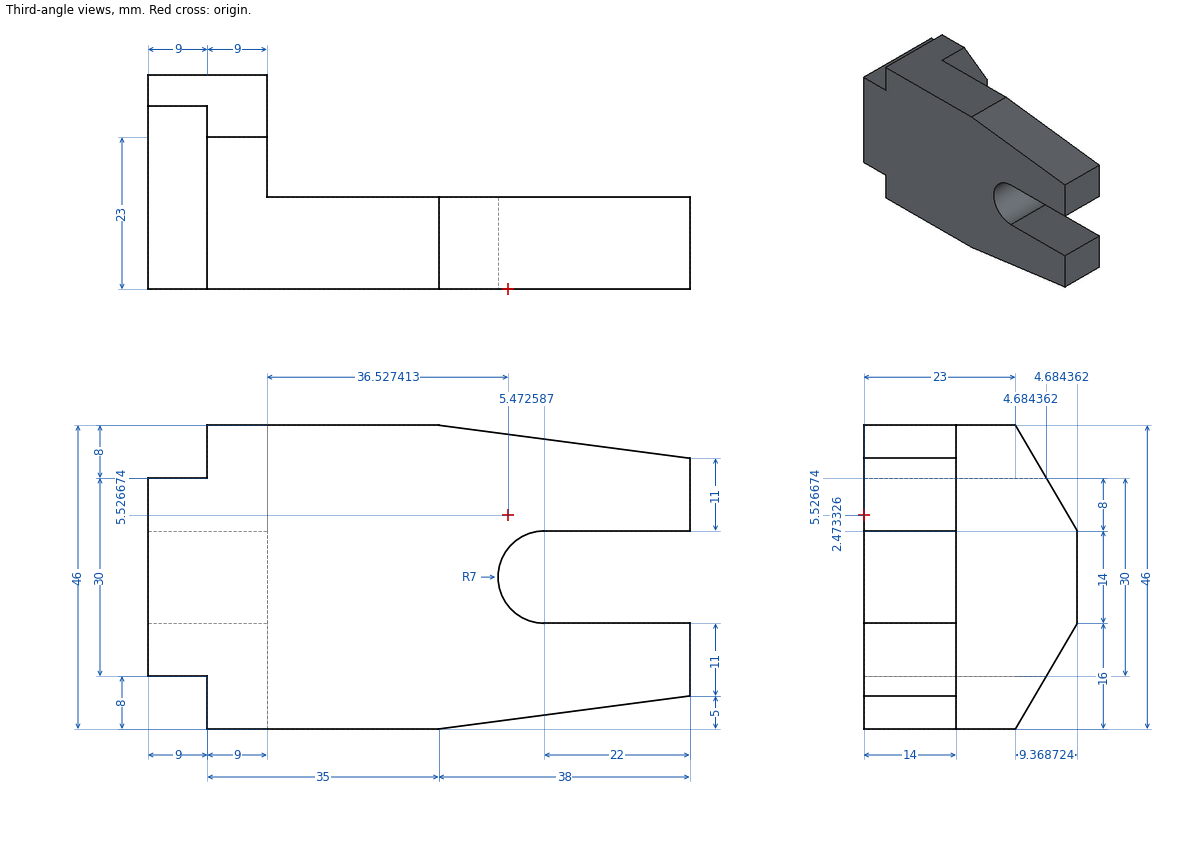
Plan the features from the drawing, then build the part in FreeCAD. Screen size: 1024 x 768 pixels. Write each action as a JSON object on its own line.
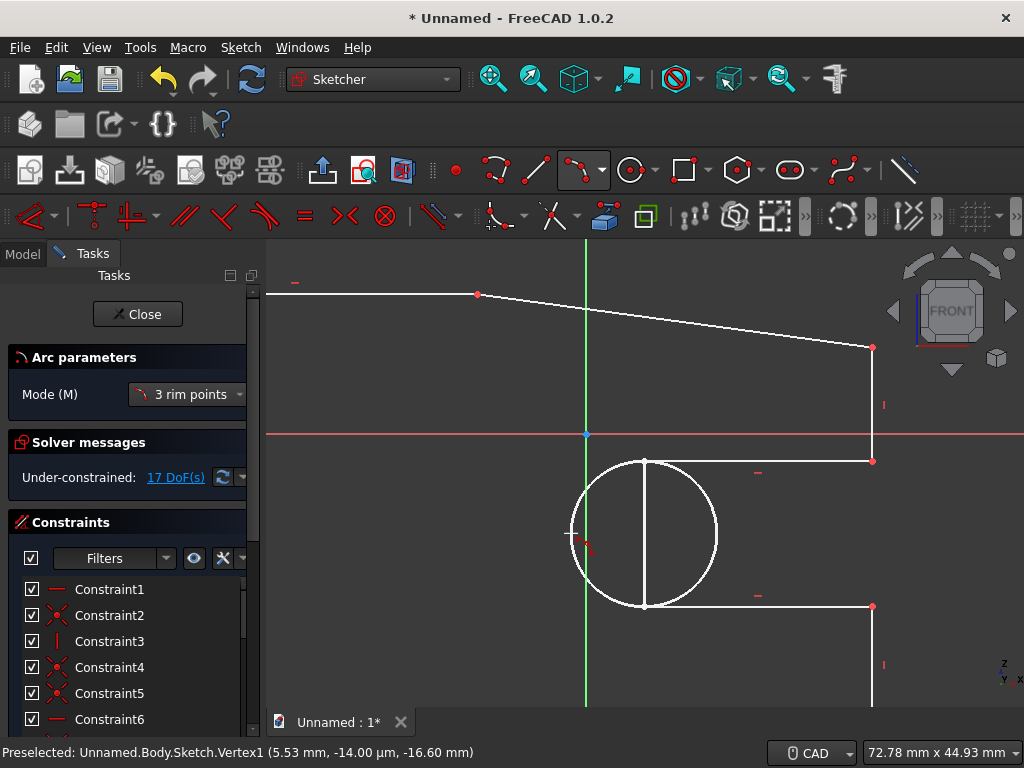
{"action": "left_click", "coordinate": [571, 533]}
{"action": "key", "text": "Escape"}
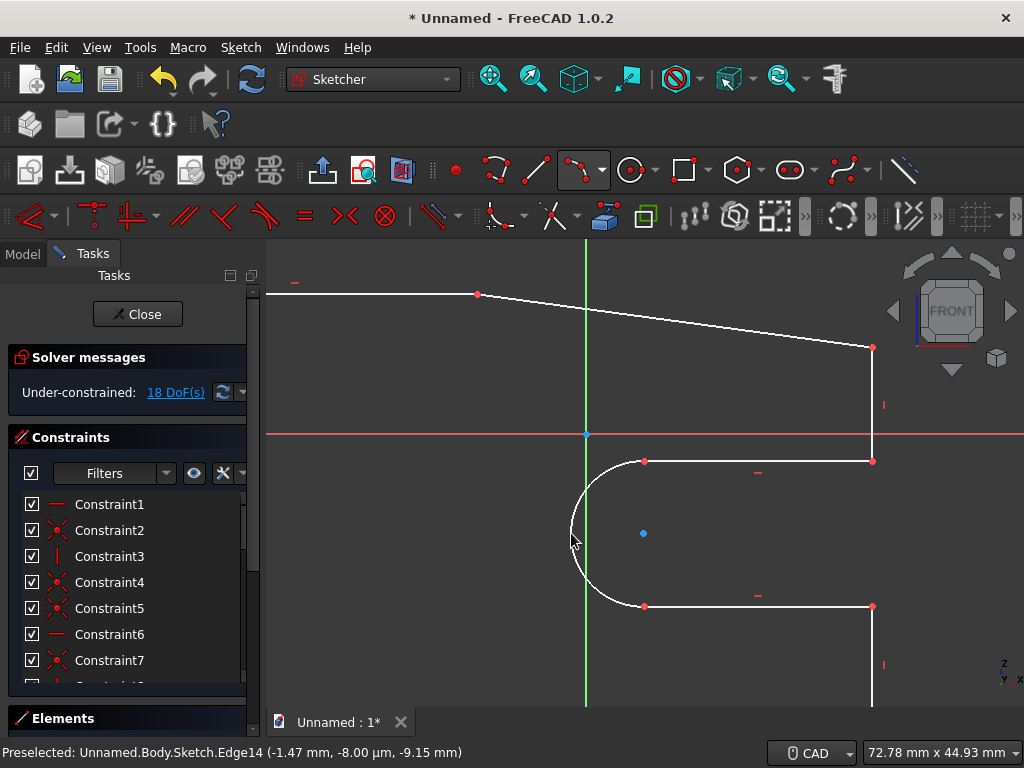
{"action": "left_click", "coordinate": [713, 607]}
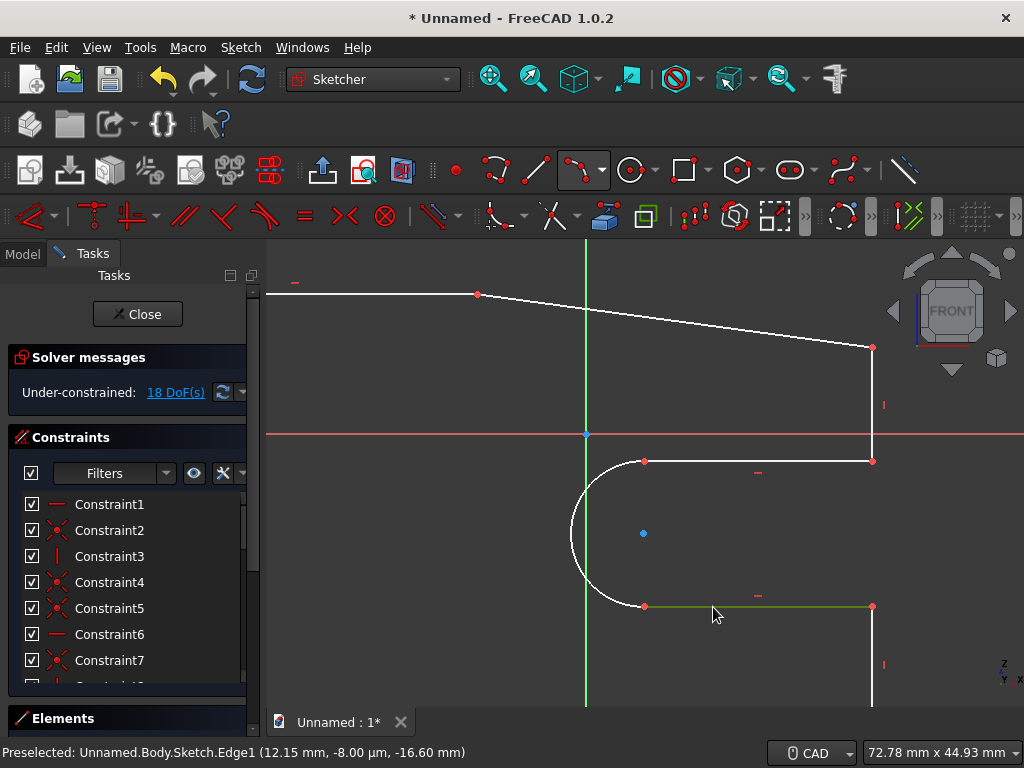
{"action": "left_click", "coordinate": [585, 491]}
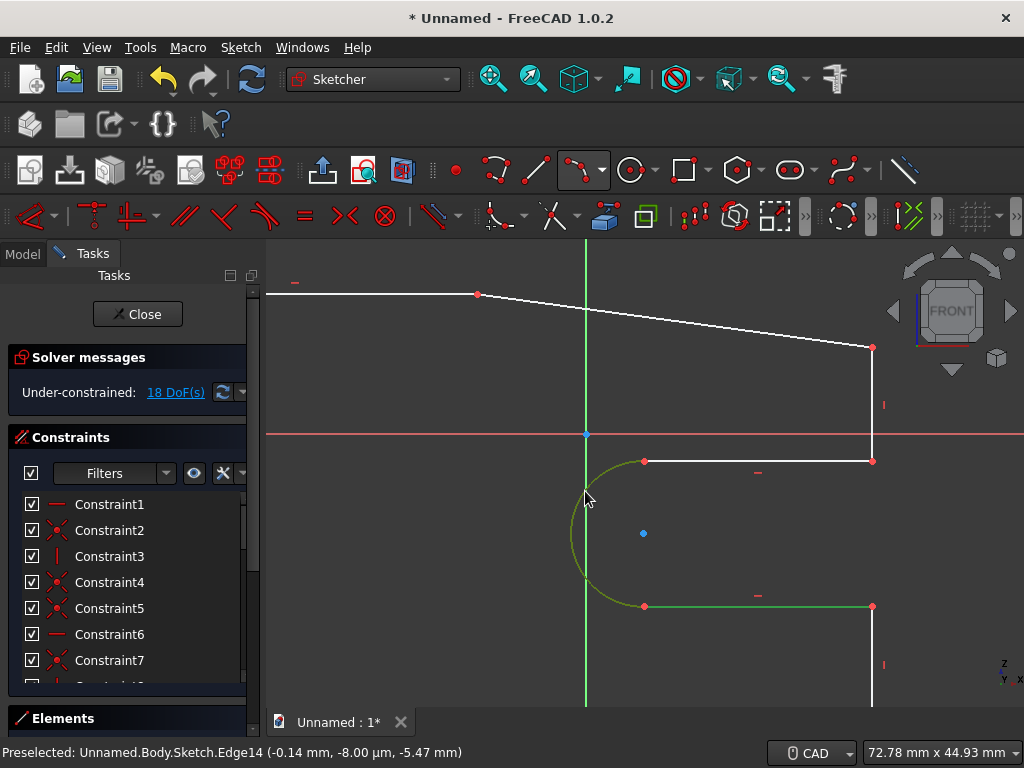
{"action": "left_click", "coordinate": [266, 216]}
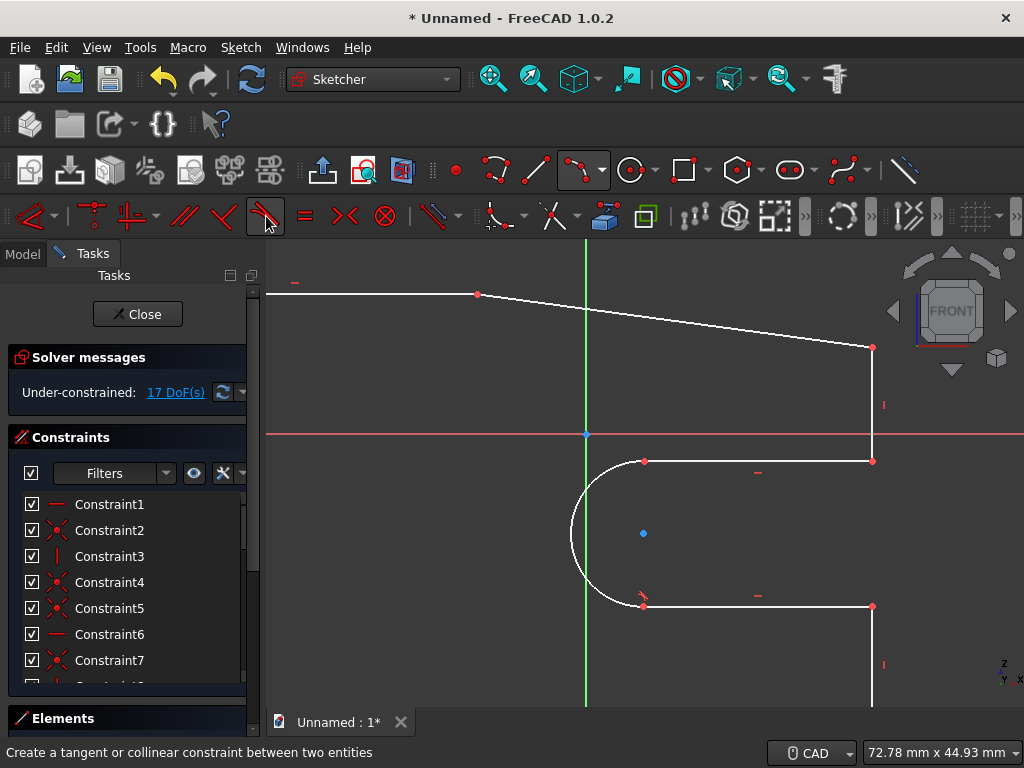
{"action": "left_click", "coordinate": [804, 461]}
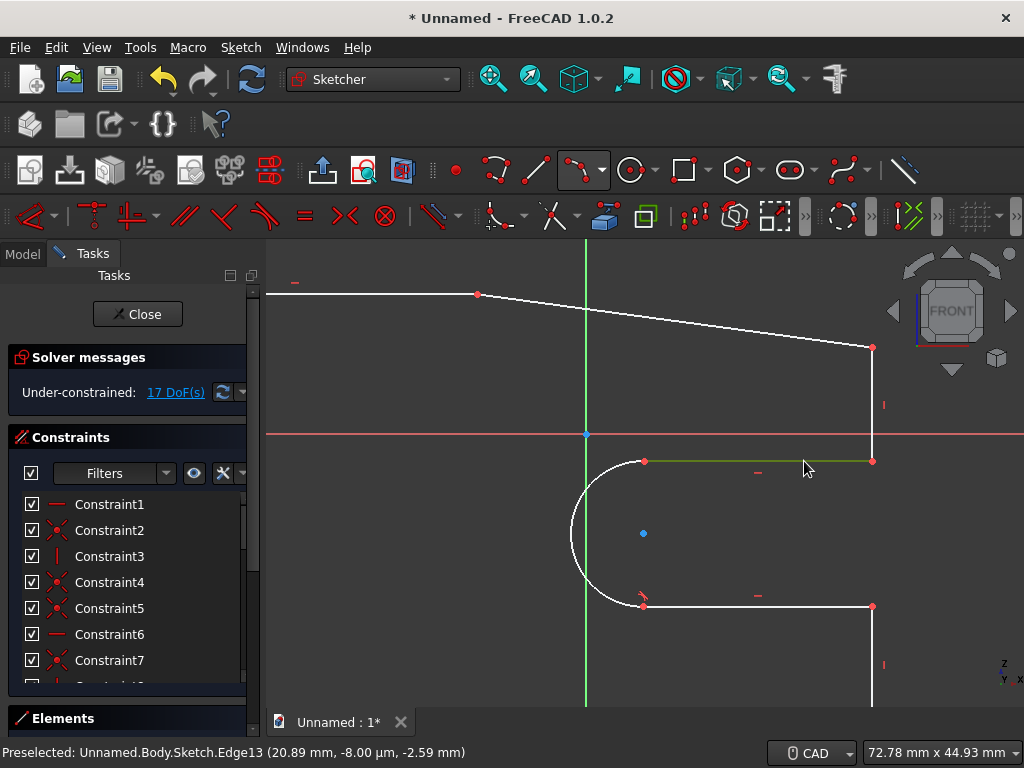
{"action": "left_click", "coordinate": [585, 491]}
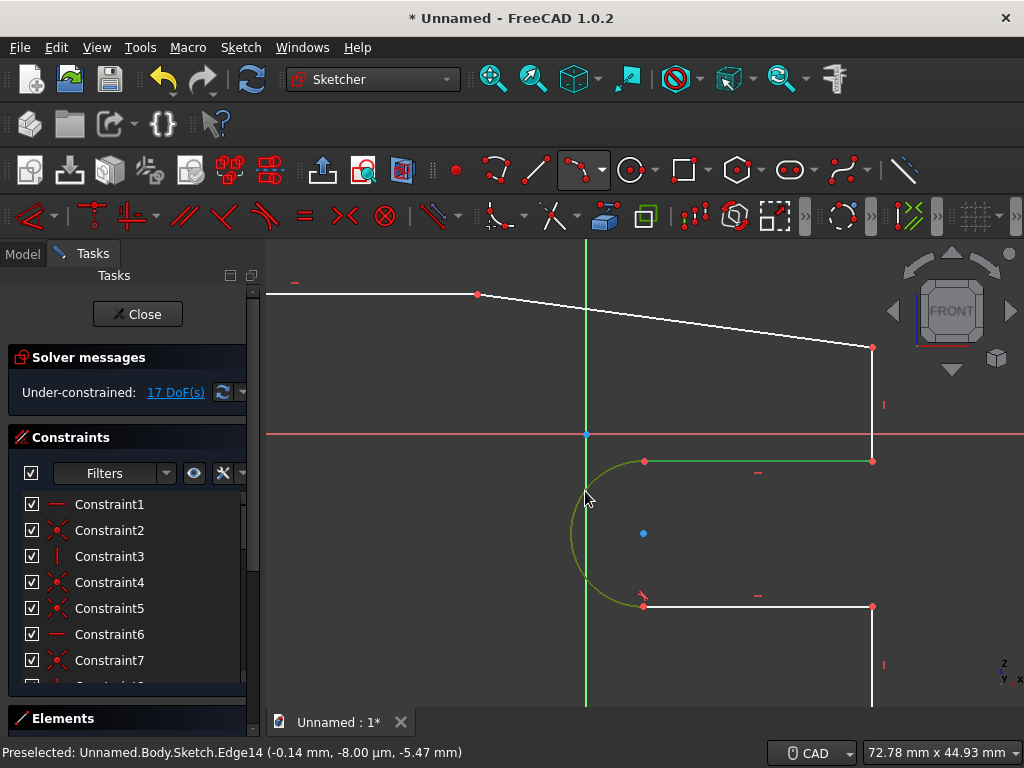
{"action": "left_click", "coordinate": [266, 216]}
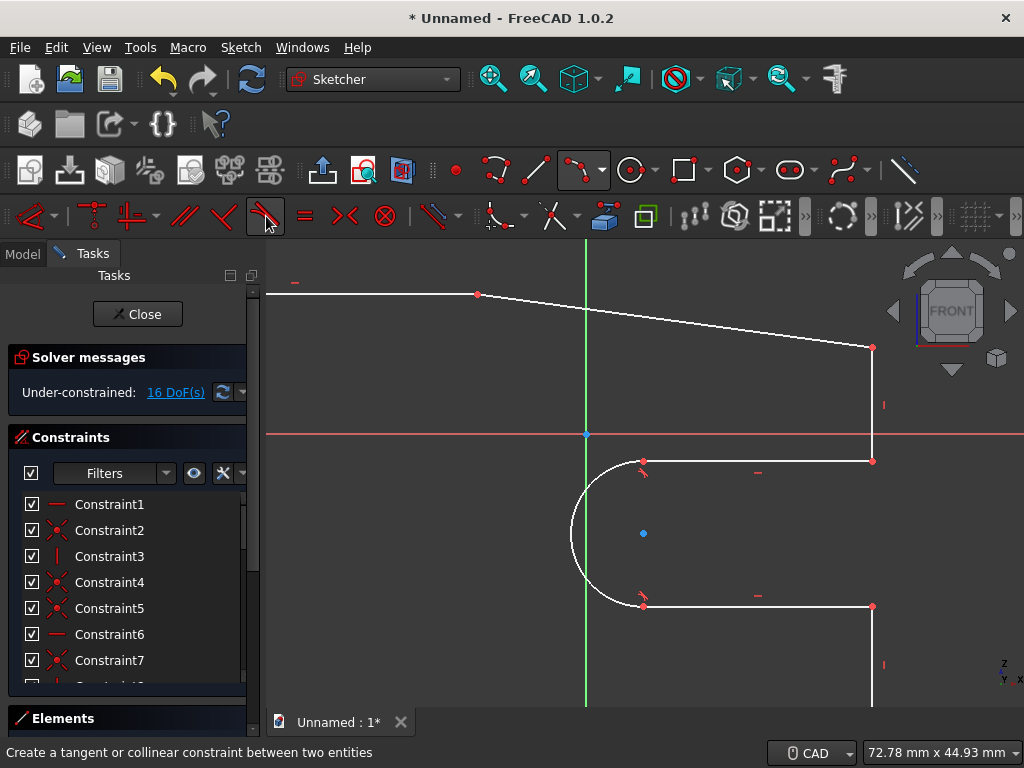
{"action": "left_click", "coordinate": [585, 491]}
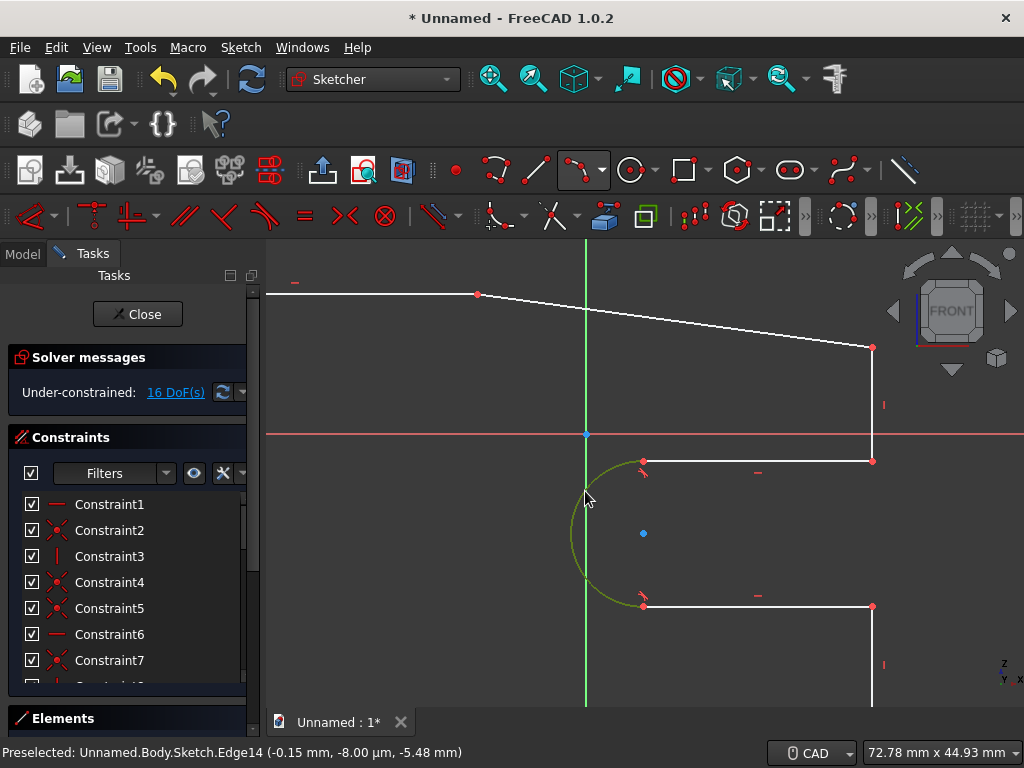
{"action": "key", "text": "k r"}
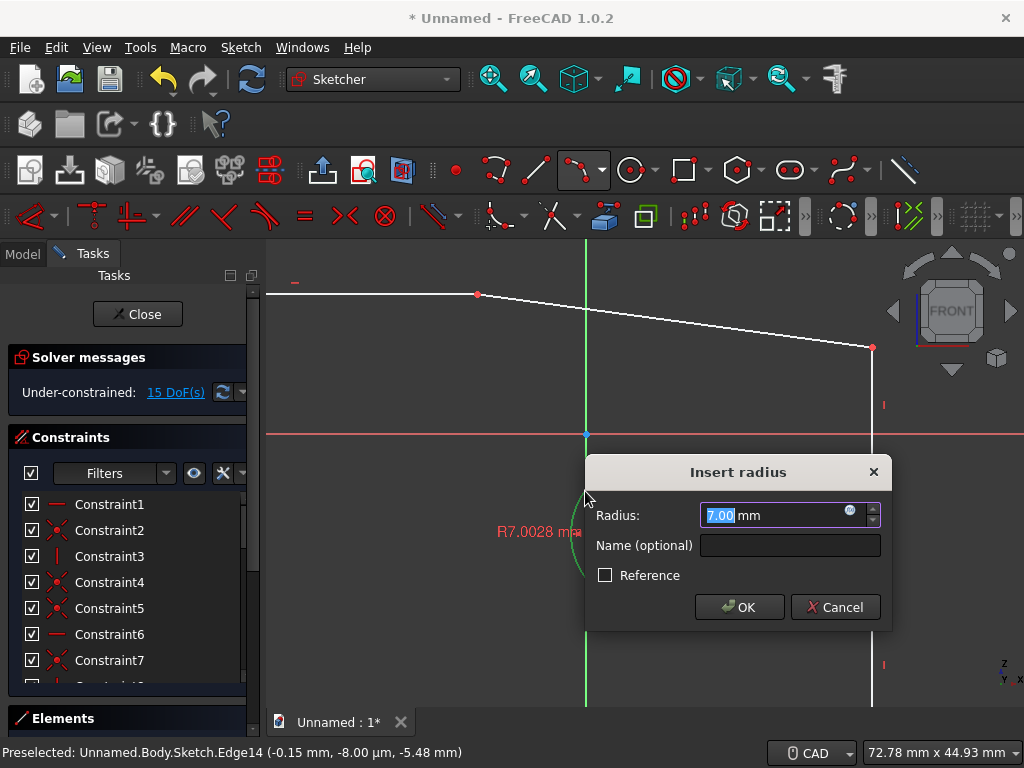
{"action": "type", "text": "7"}
{"action": "key", "text": "Return"}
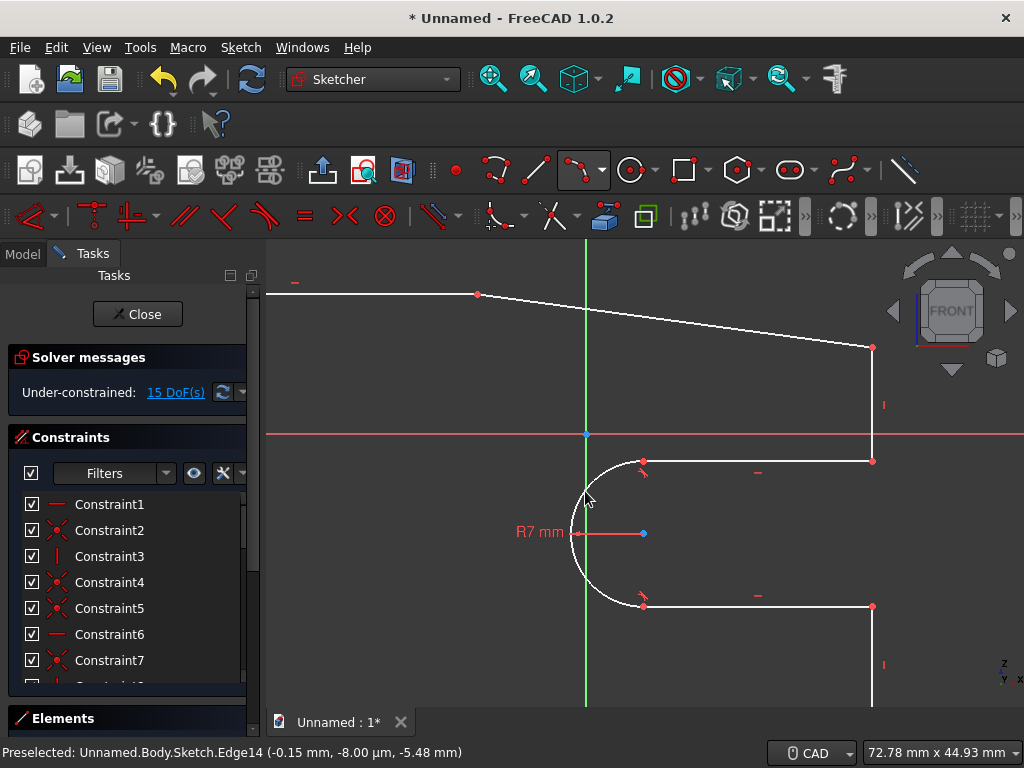
{"action": "scroll", "coordinate": [683, 424], "scroll_direction": "down", "scroll_amount": 4}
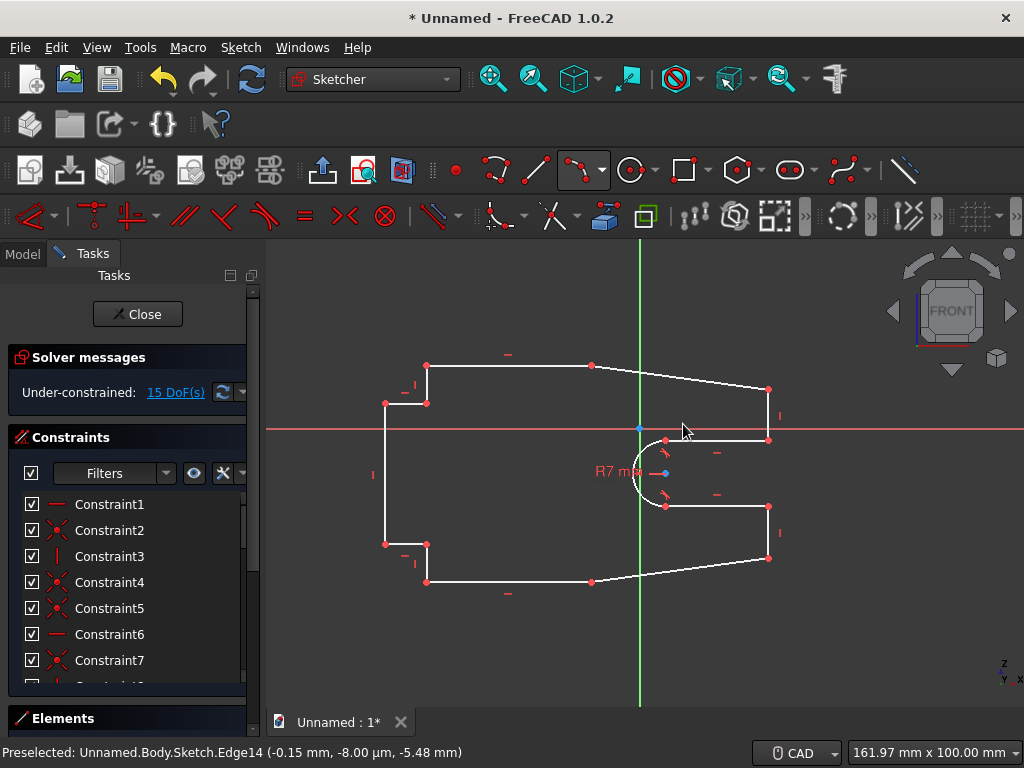
{"action": "left_click", "coordinate": [427, 571]}